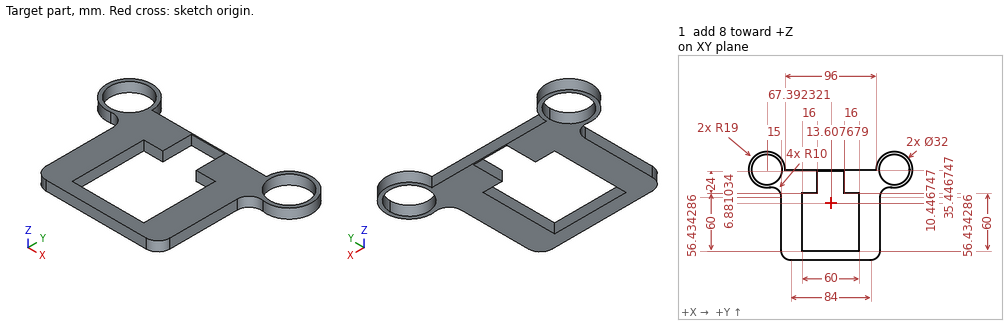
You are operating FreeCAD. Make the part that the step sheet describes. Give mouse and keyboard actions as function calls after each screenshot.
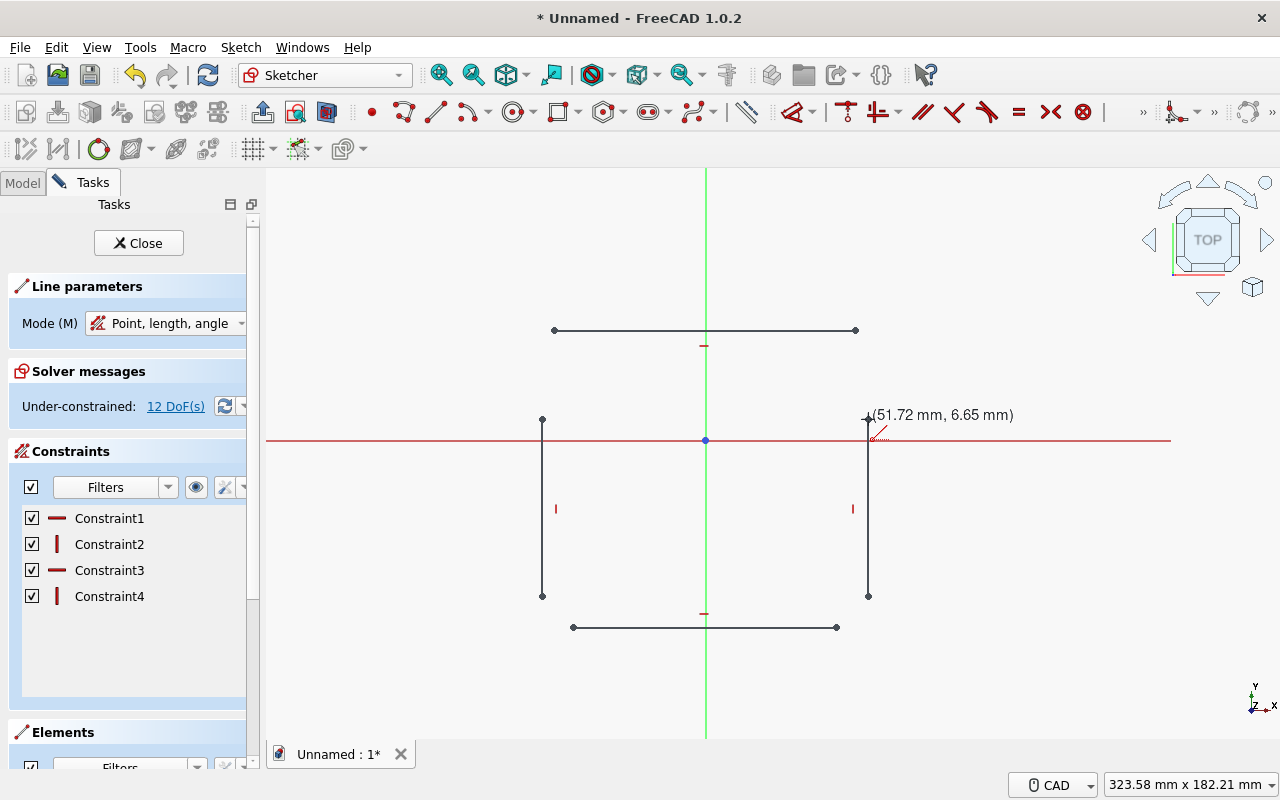
key(g)
key(3)
key(a)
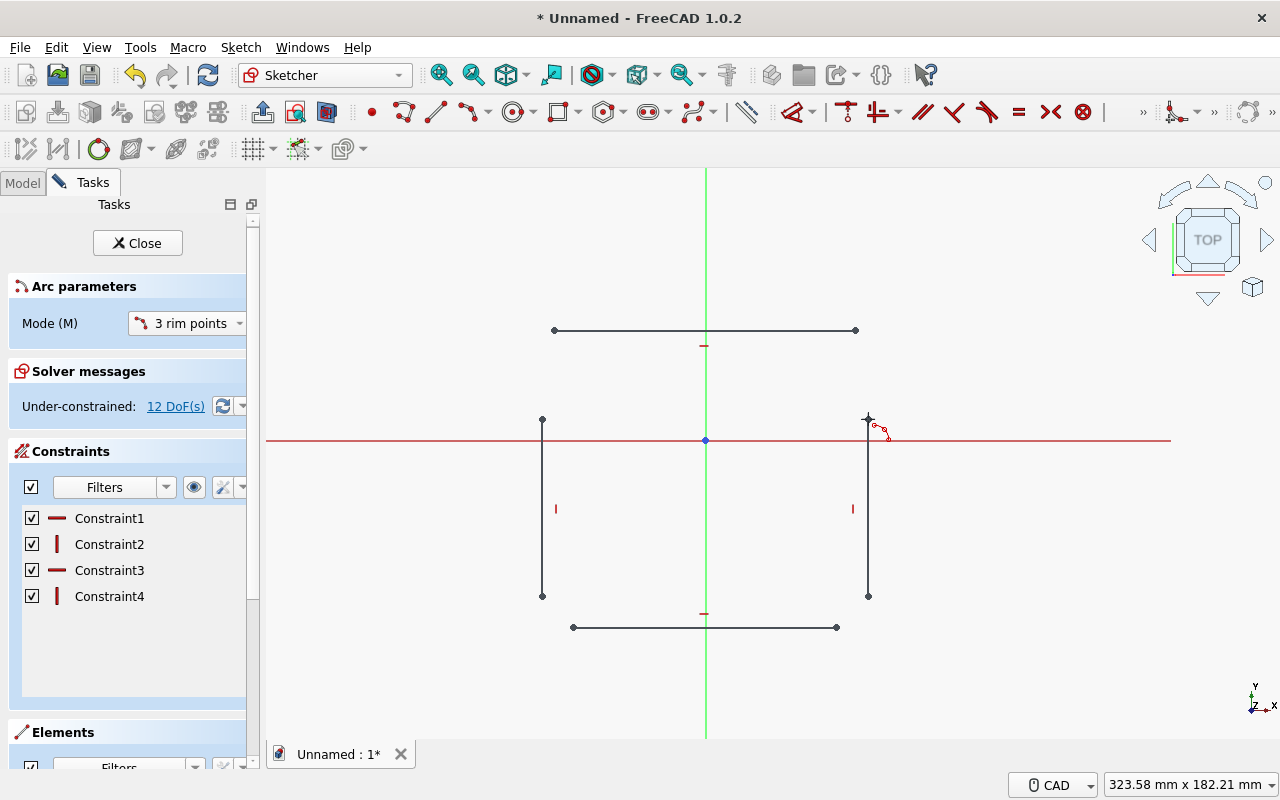
click(554, 331)
click(505, 388)
click(449, 291)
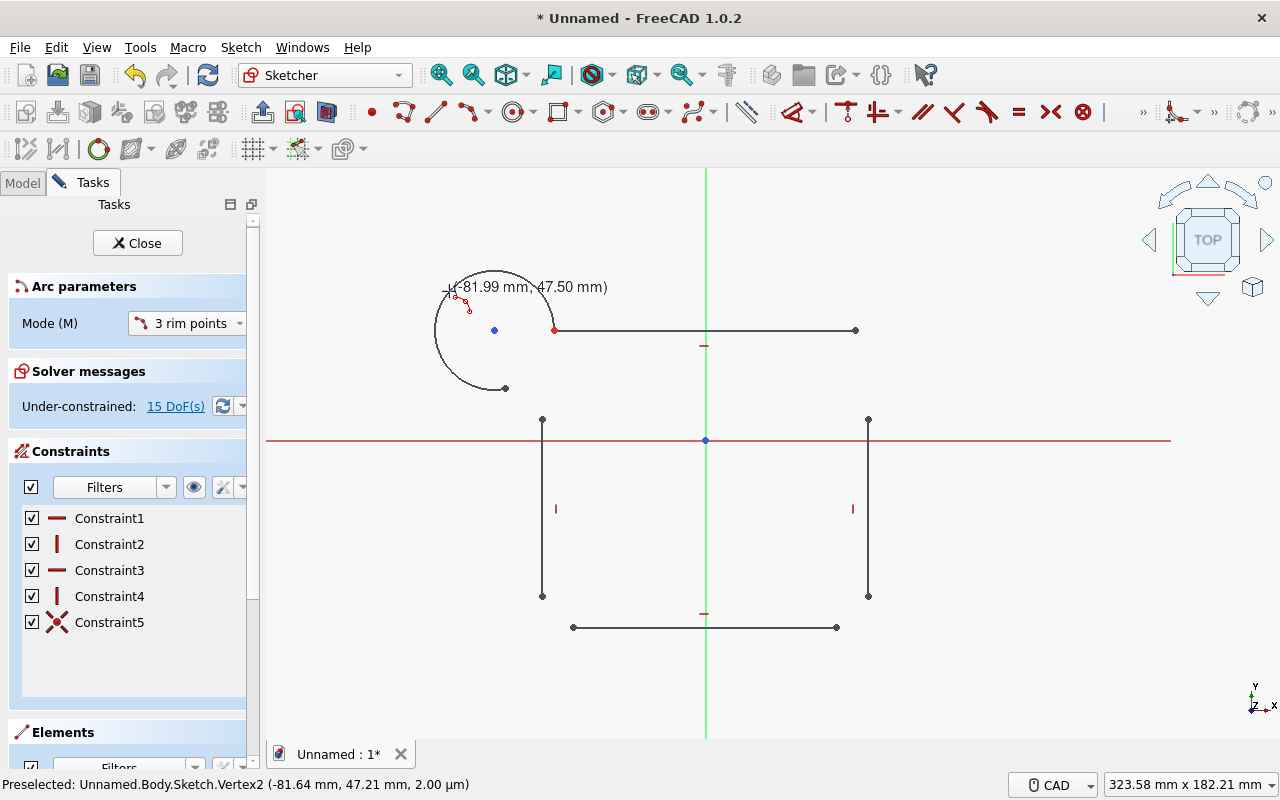
click(505, 389)
click(542, 420)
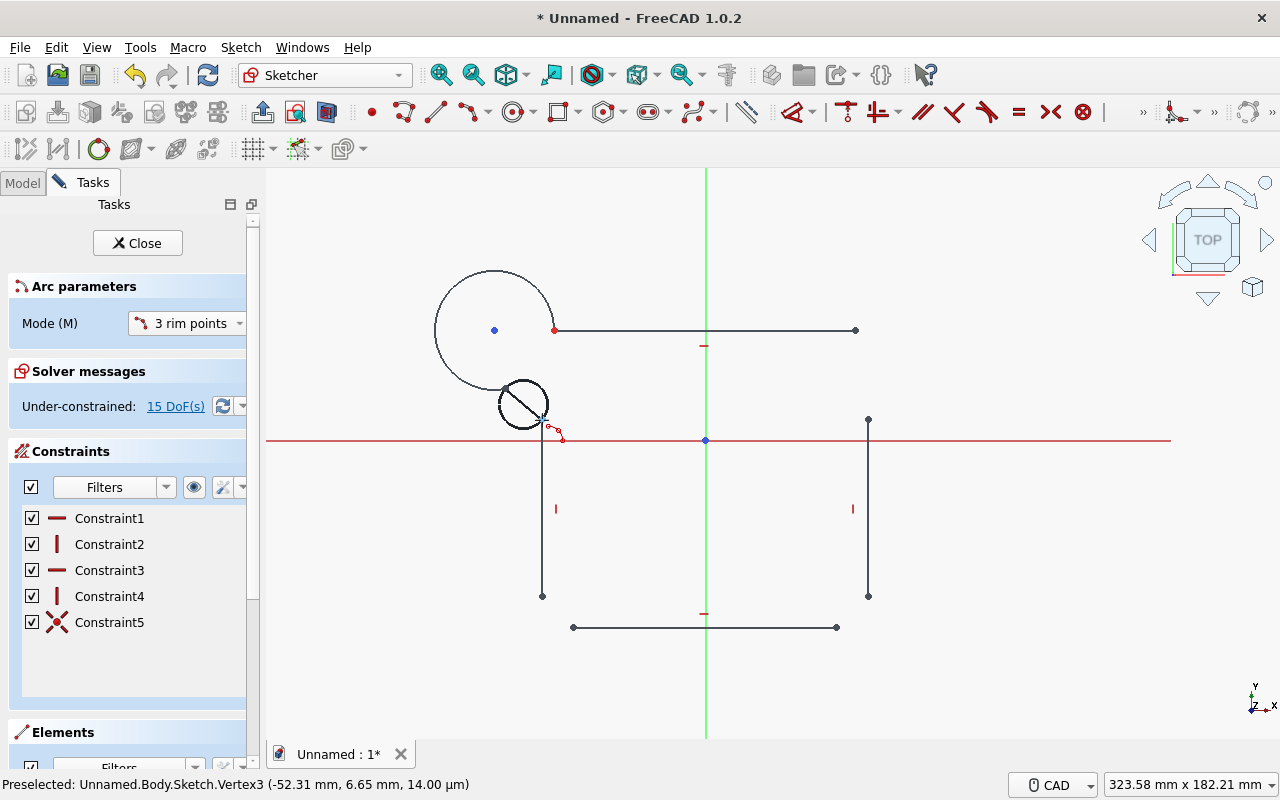
scroll(531, 395, up, 2)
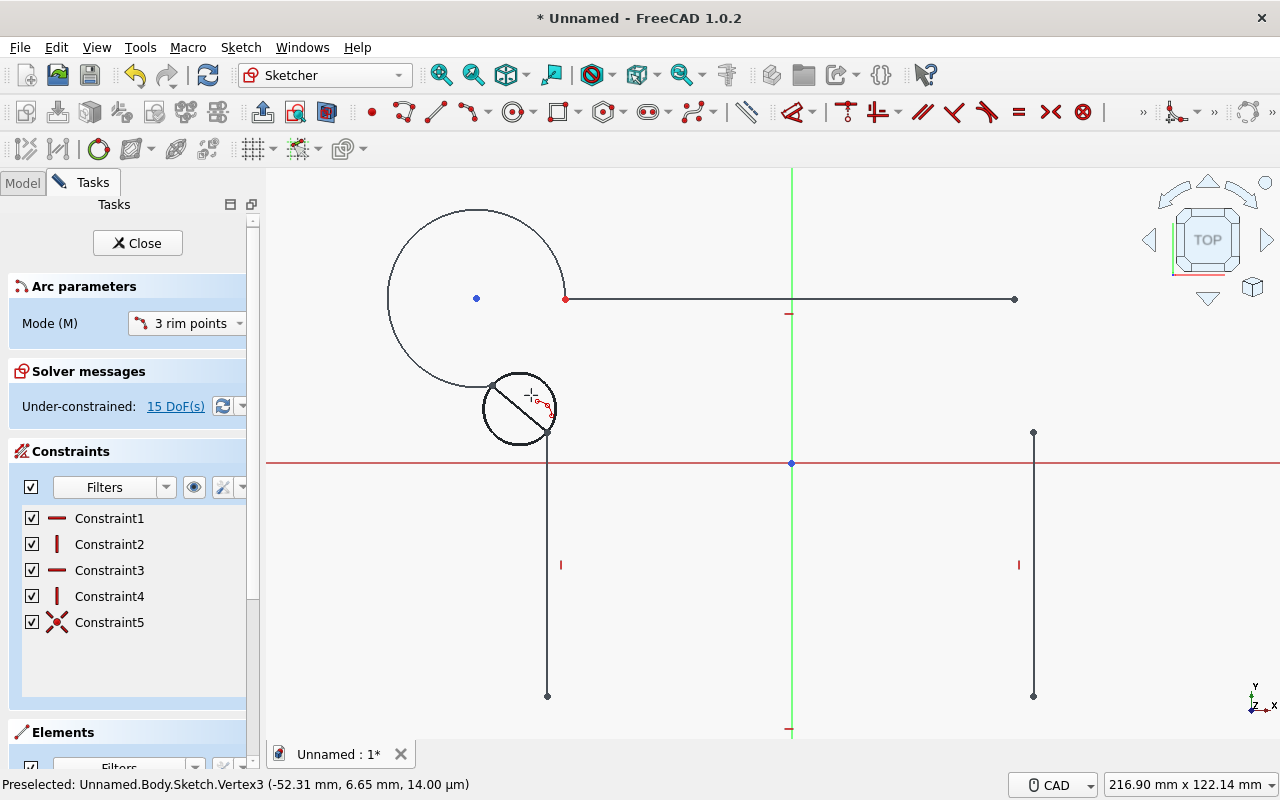
click(530, 395)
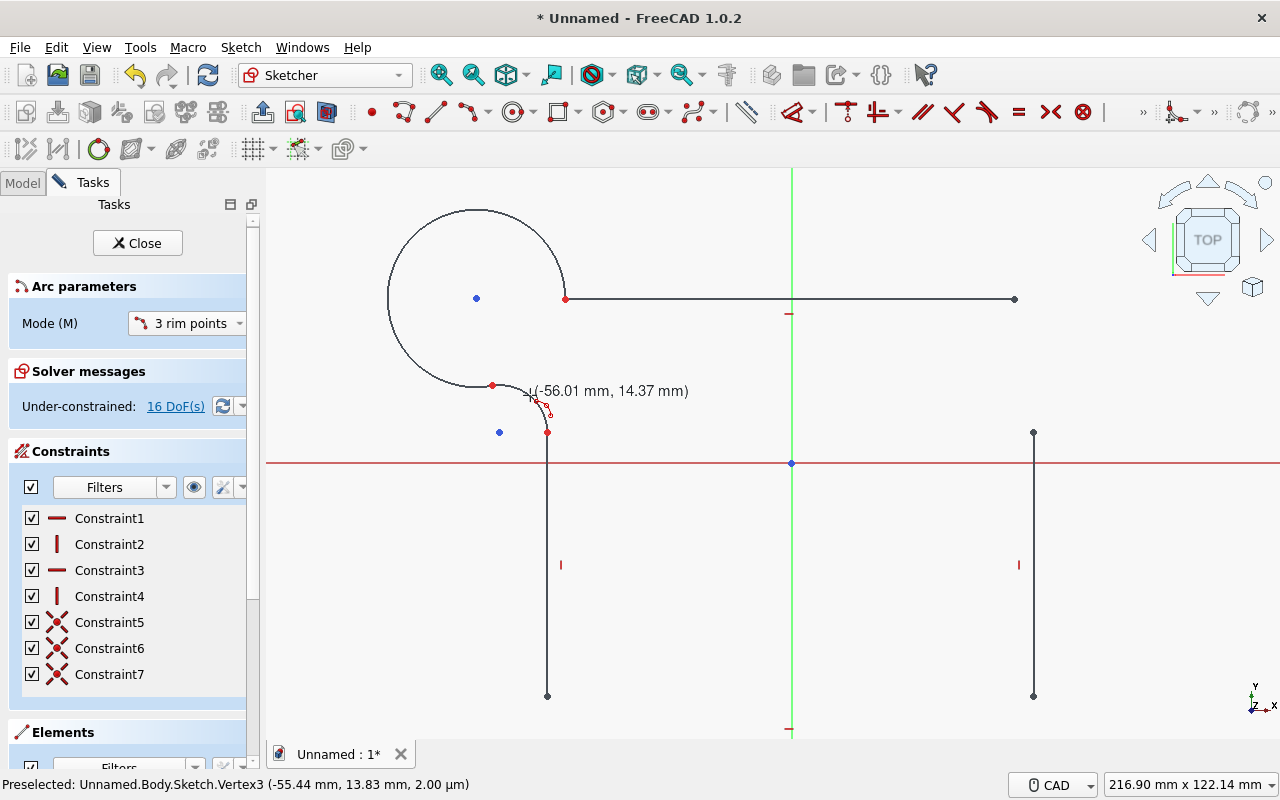
click(547, 696)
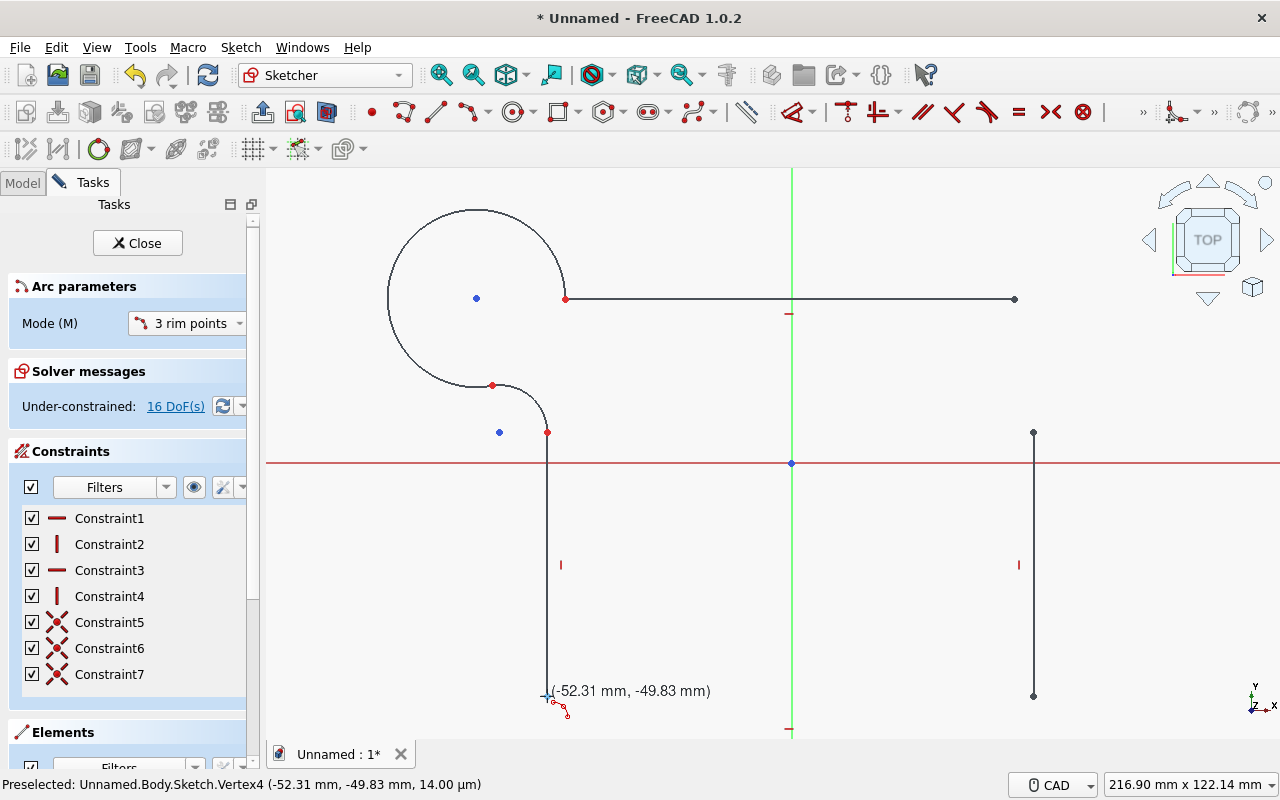
scroll(531, 395, down, 2)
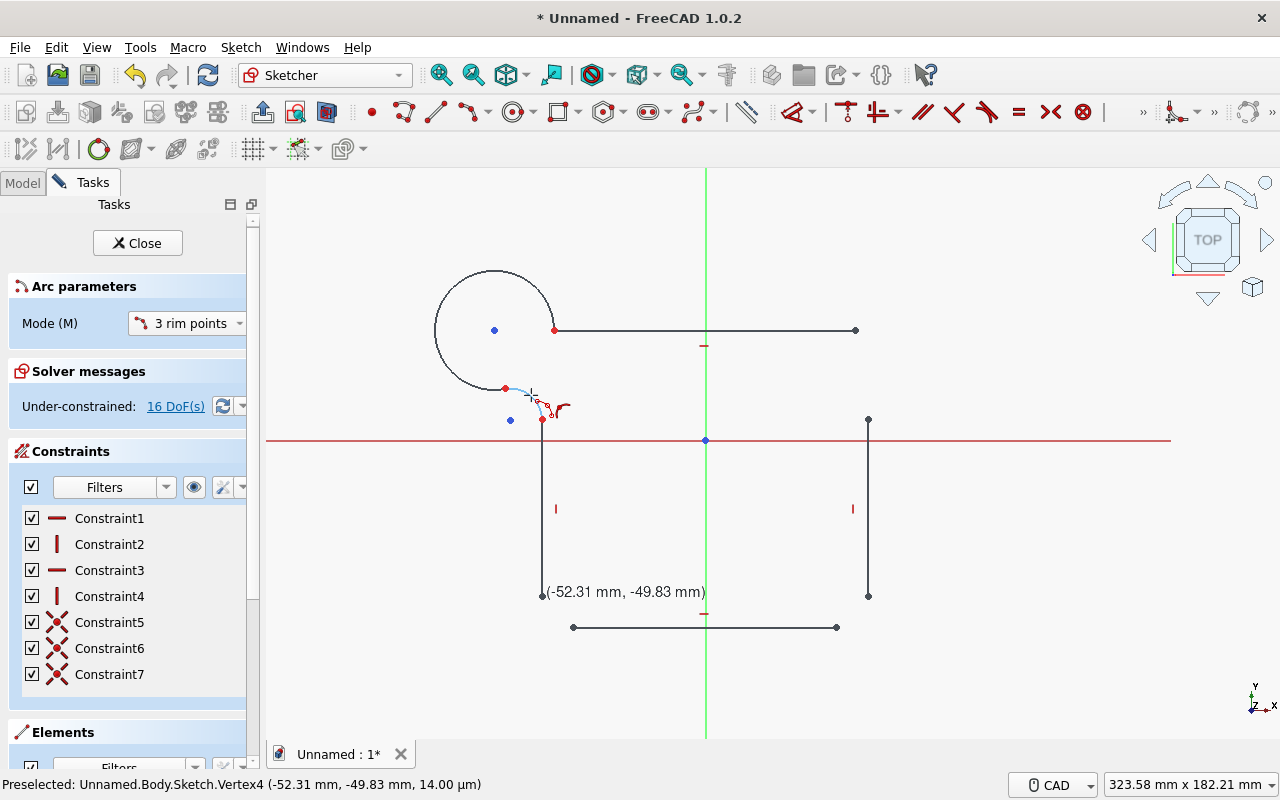
click(573, 628)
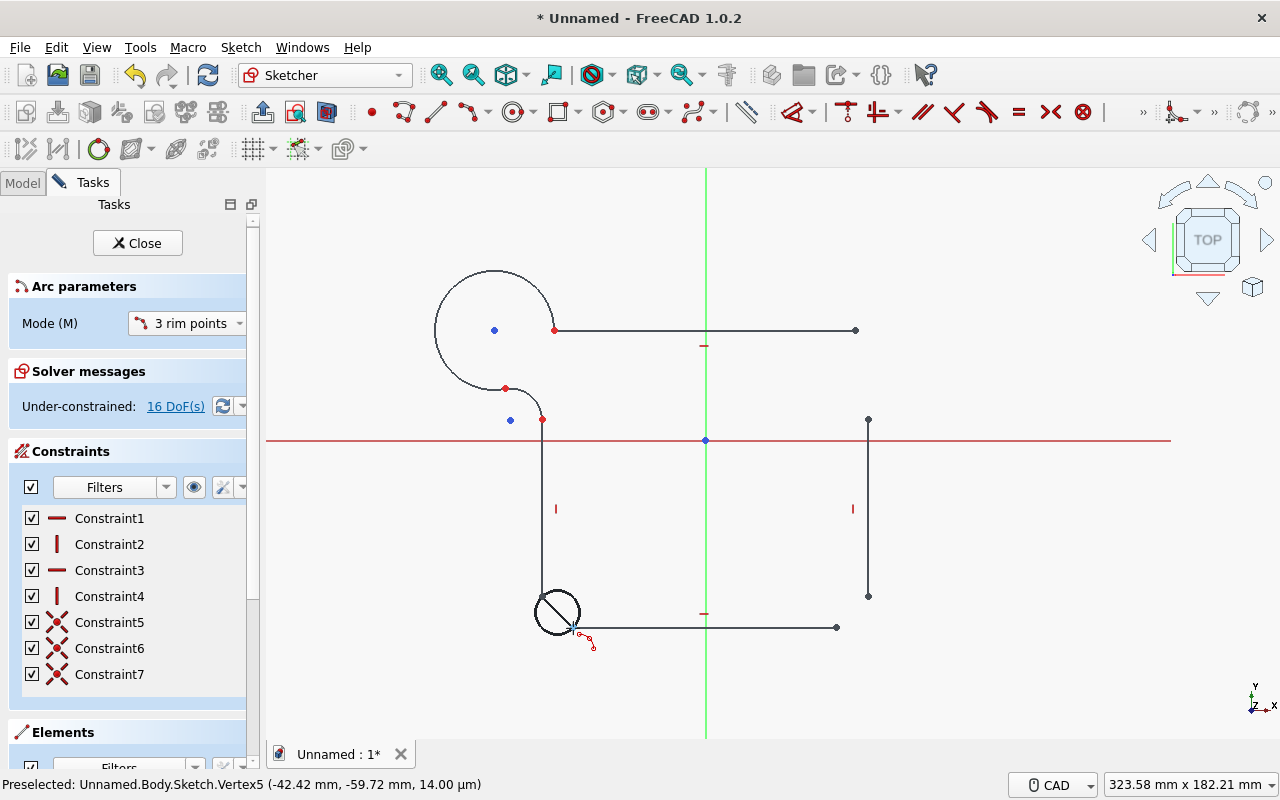
scroll(551, 618, up, 3)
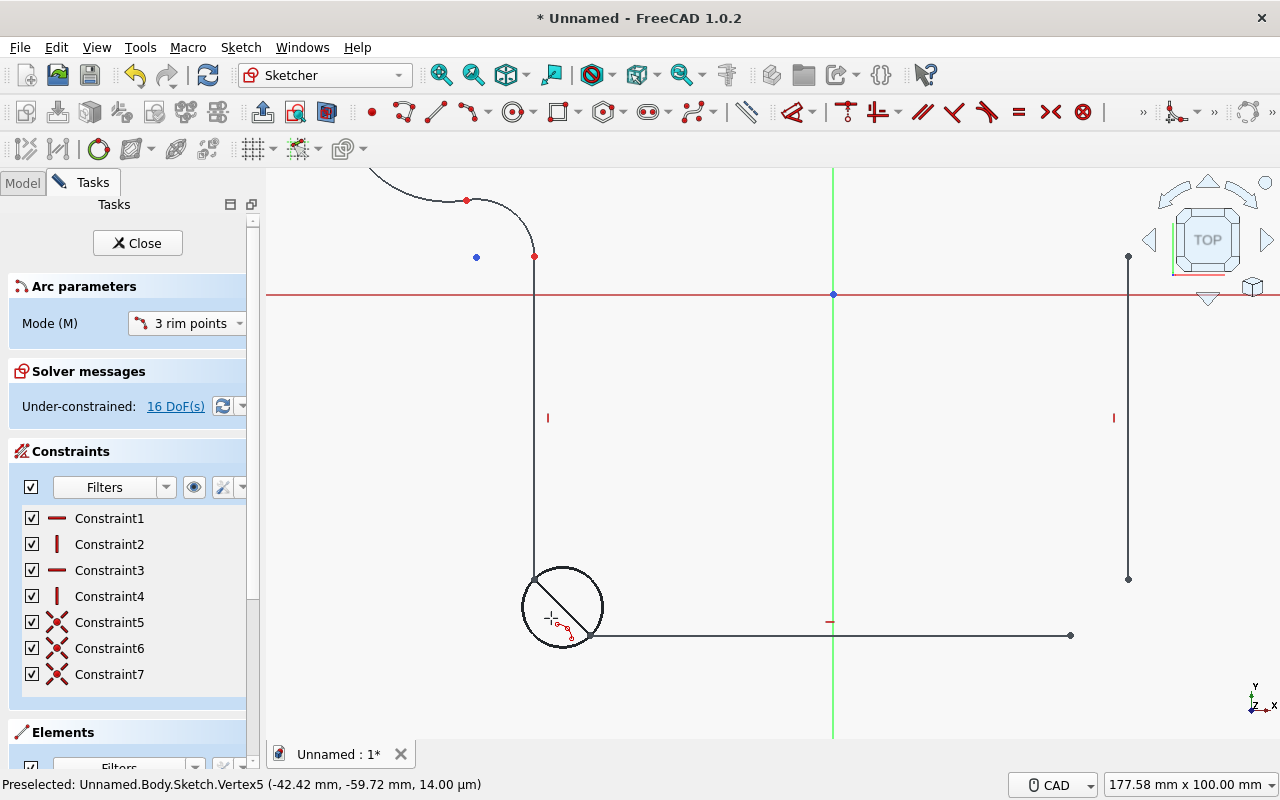
click(551, 618)